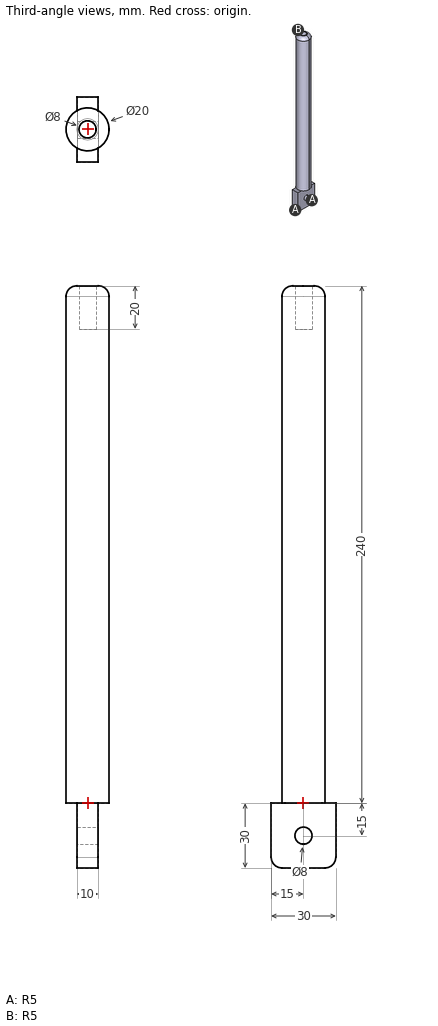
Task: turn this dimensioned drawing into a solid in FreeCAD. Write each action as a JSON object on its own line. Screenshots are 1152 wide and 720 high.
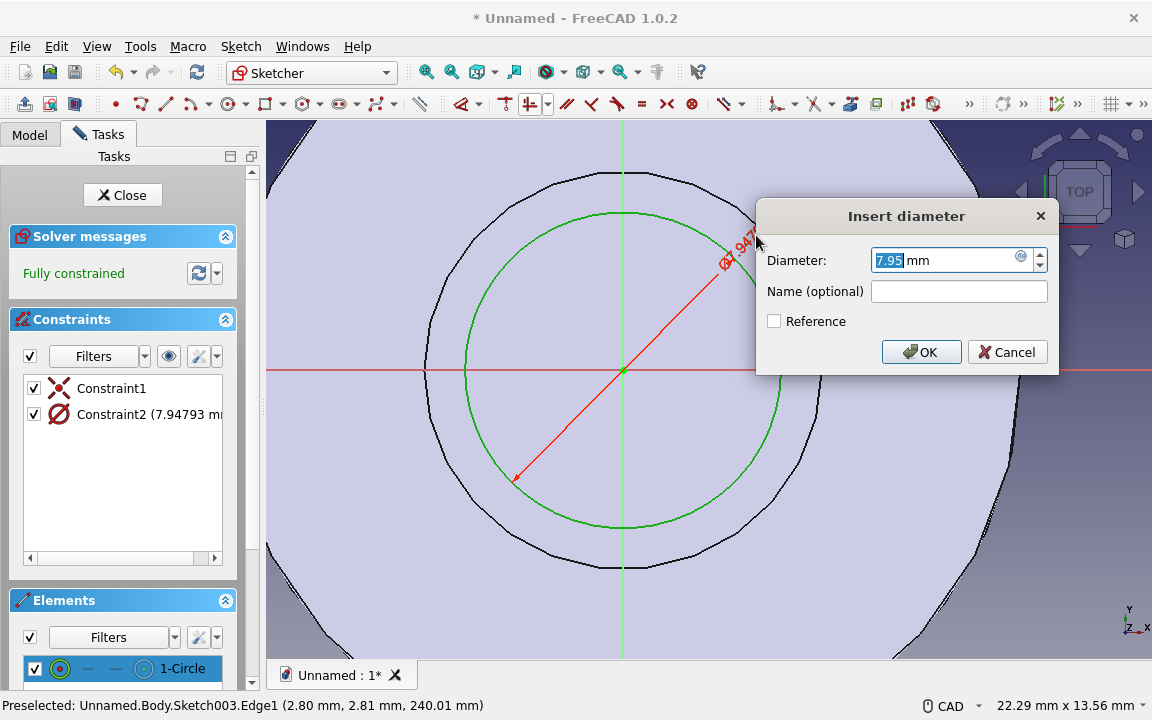
{"action": "type", "text": "8"}
{"action": "key", "text": "Return"}
{"action": "key", "text": "Escape"}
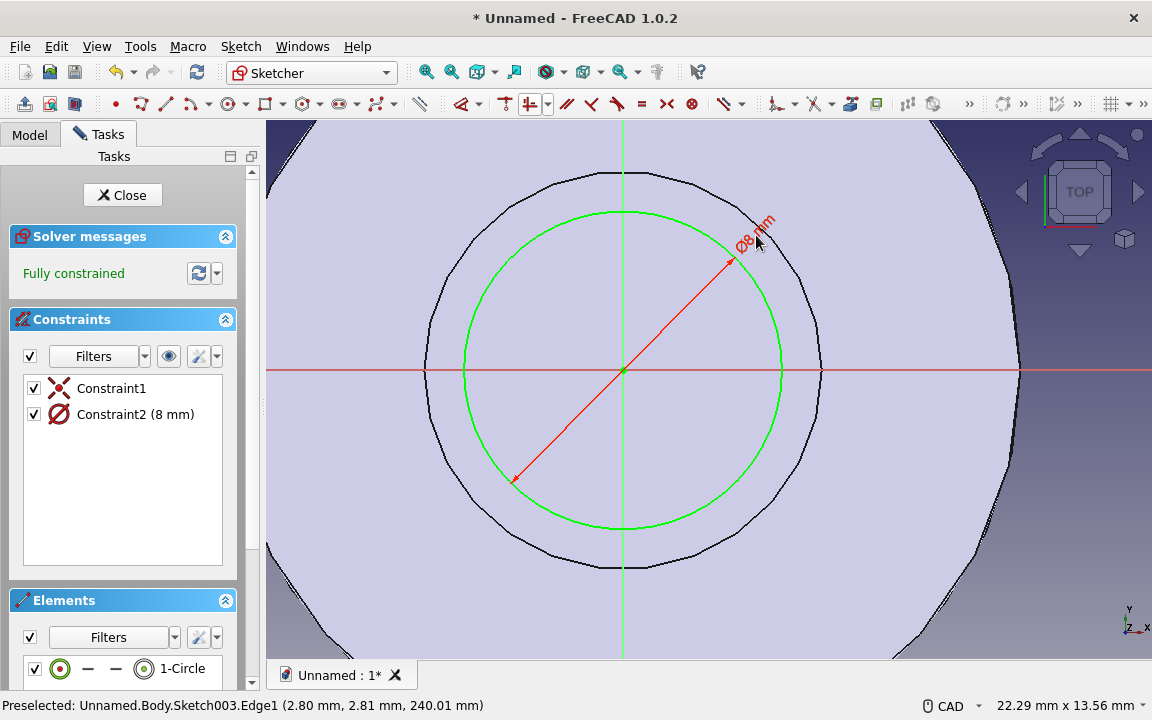
{"action": "left_click", "coordinate": [123, 195]}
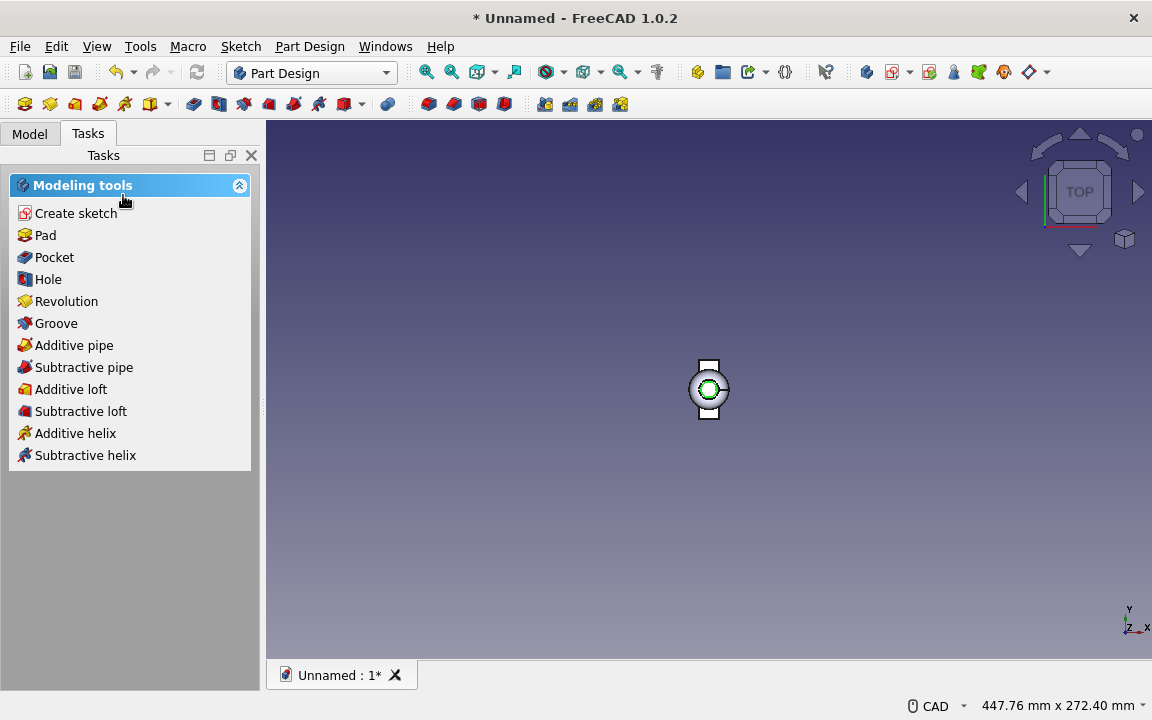
{"action": "left_click", "coordinate": [194, 104]}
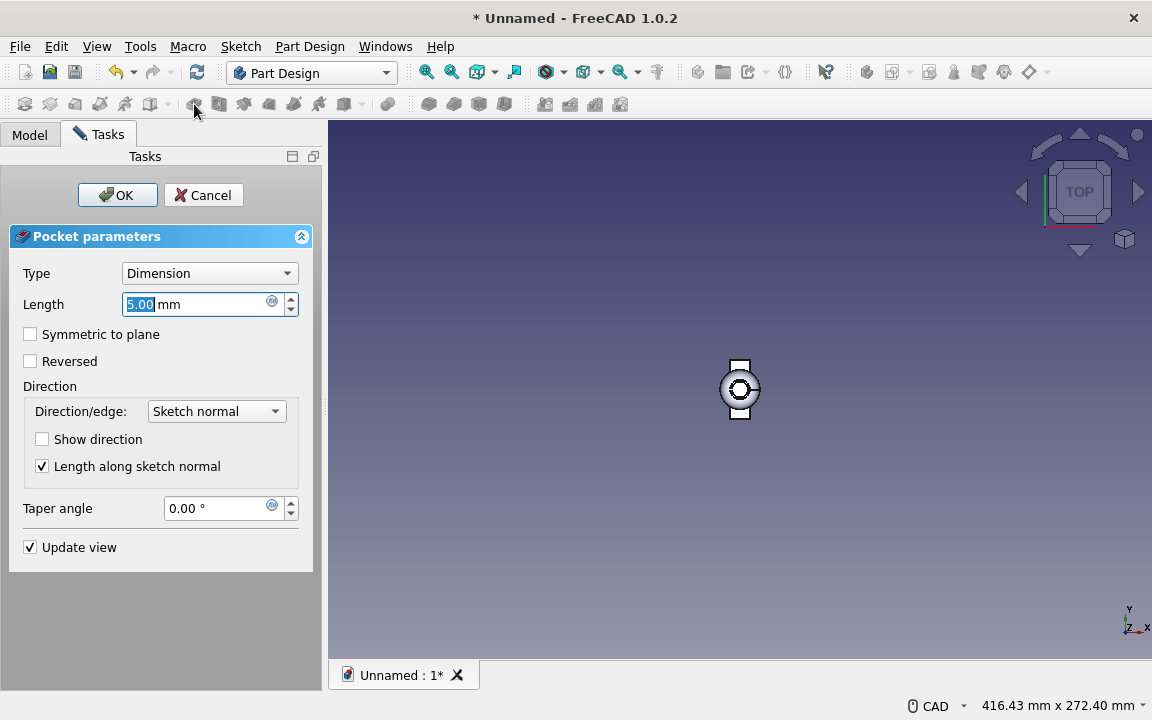
{"action": "type", "text": "20"}
{"action": "key", "text": "Tab"}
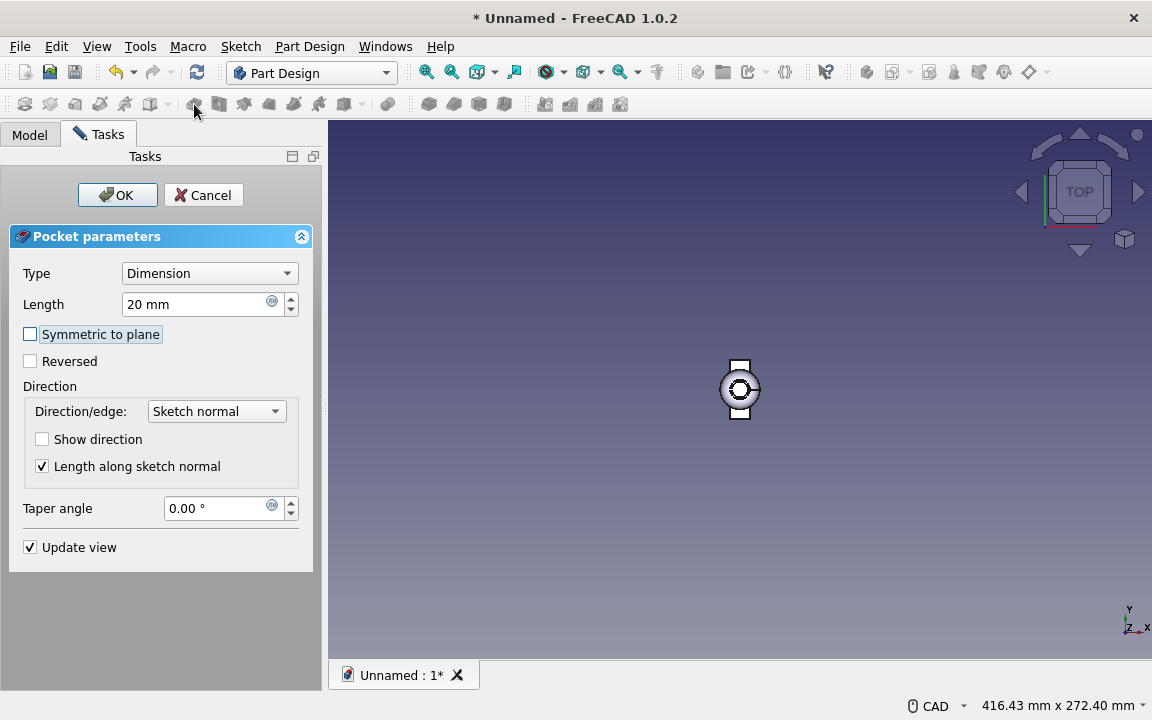
{"action": "left_click", "coordinate": [118, 195]}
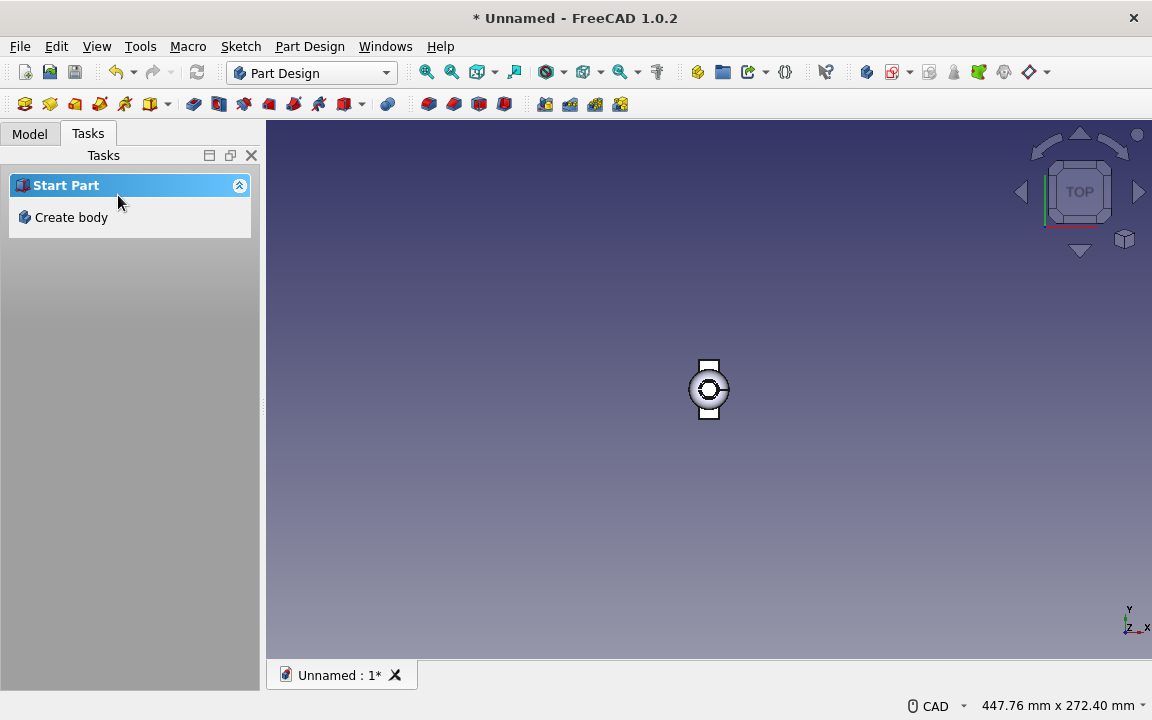
{"action": "key", "text": "0"}